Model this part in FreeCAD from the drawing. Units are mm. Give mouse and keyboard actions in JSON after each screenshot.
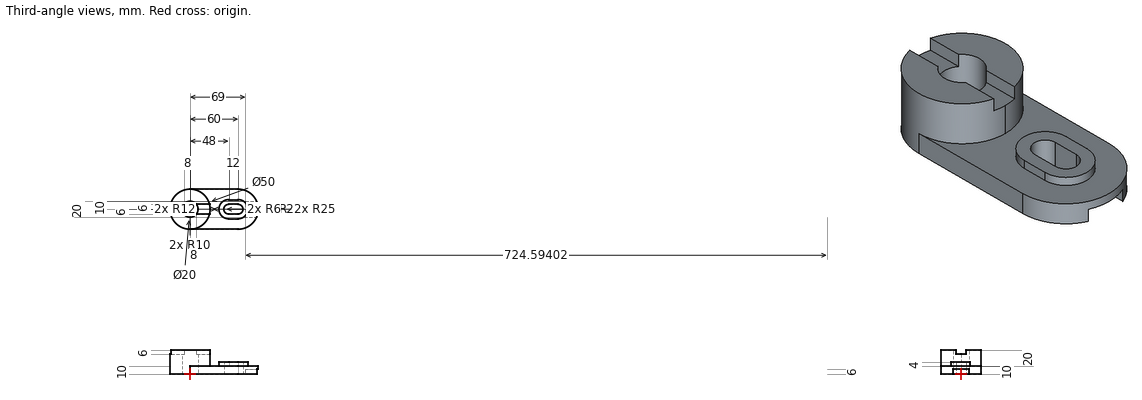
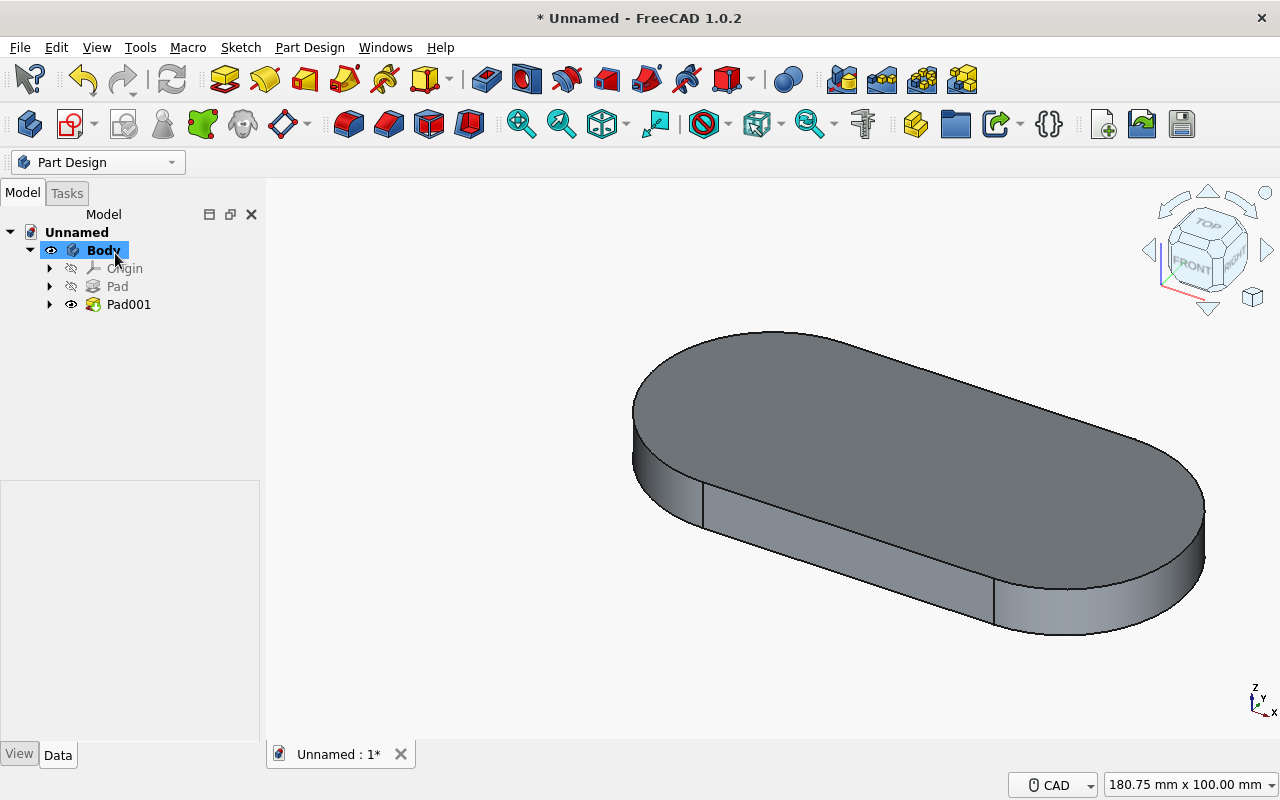
{"action": "left_click", "coordinate": [50, 268]}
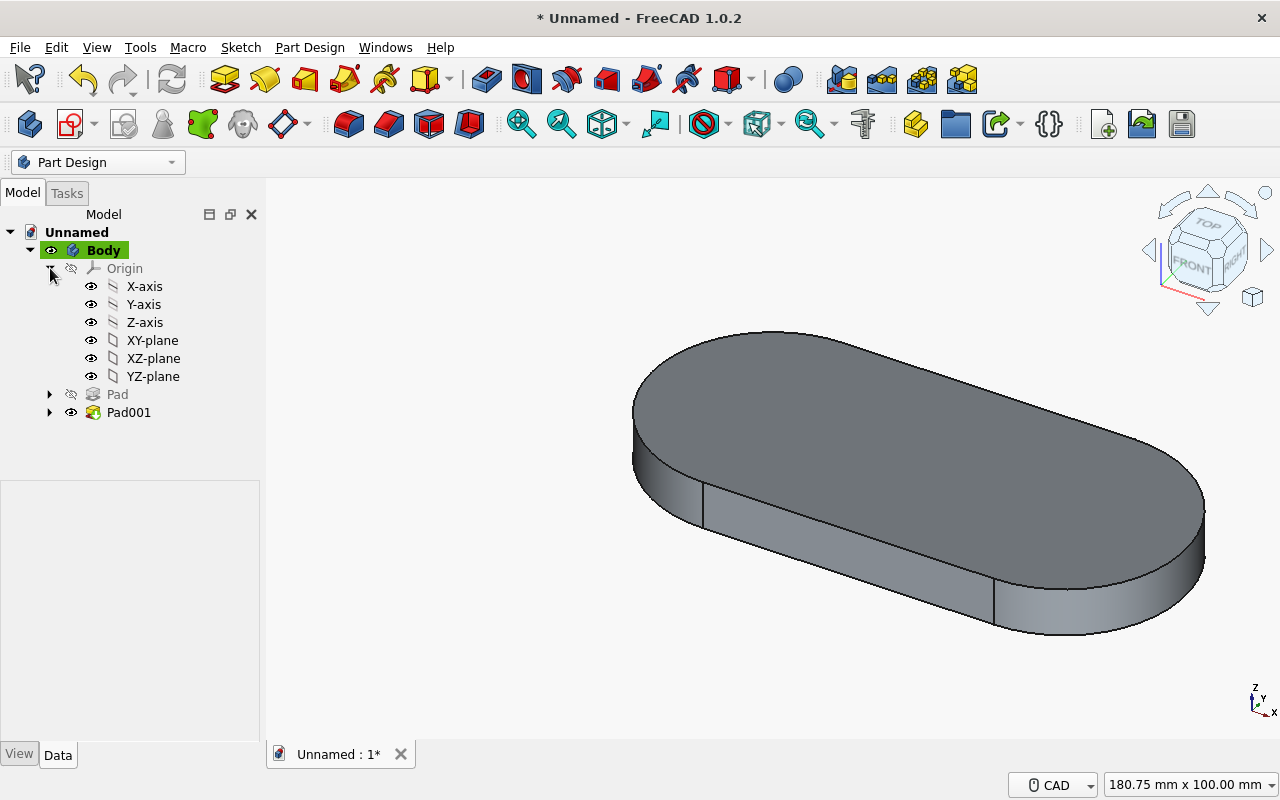
{"action": "left_click", "coordinate": [136, 340]}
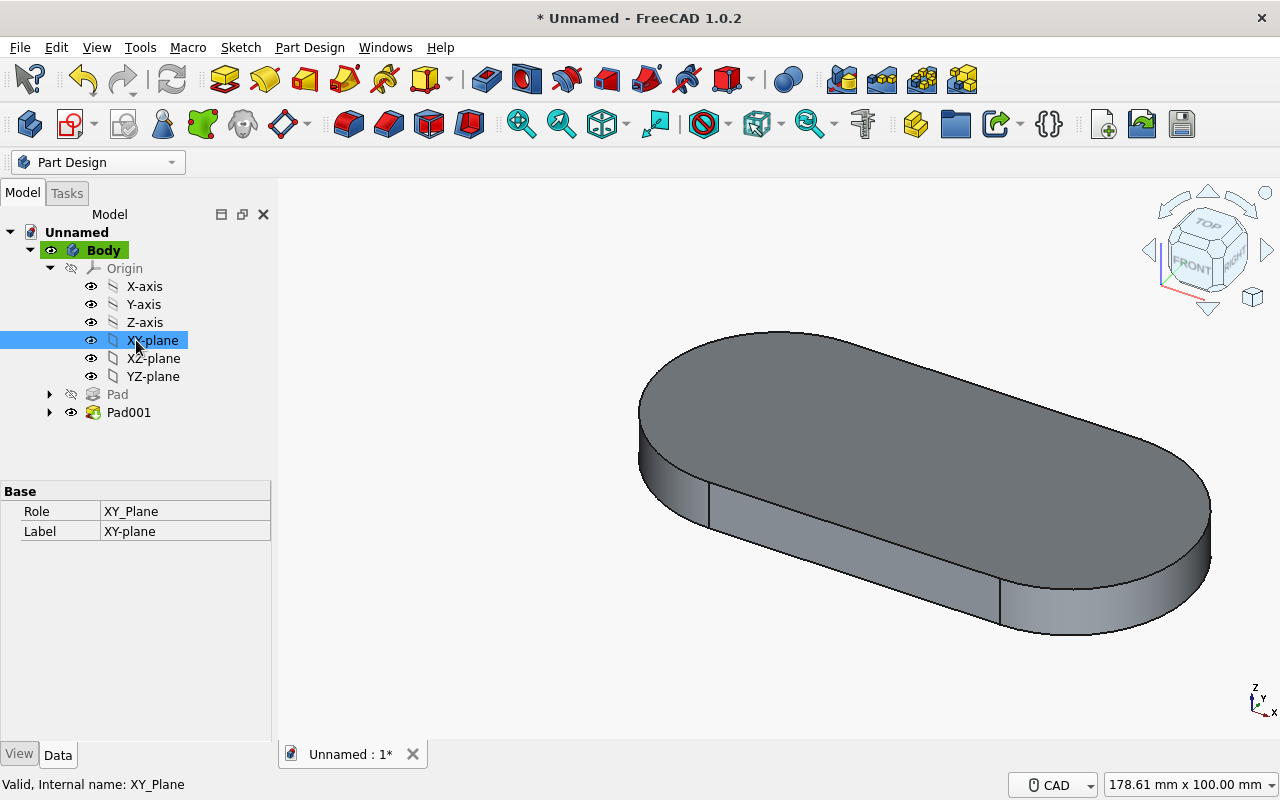
{"action": "left_click", "coordinate": [284, 124]}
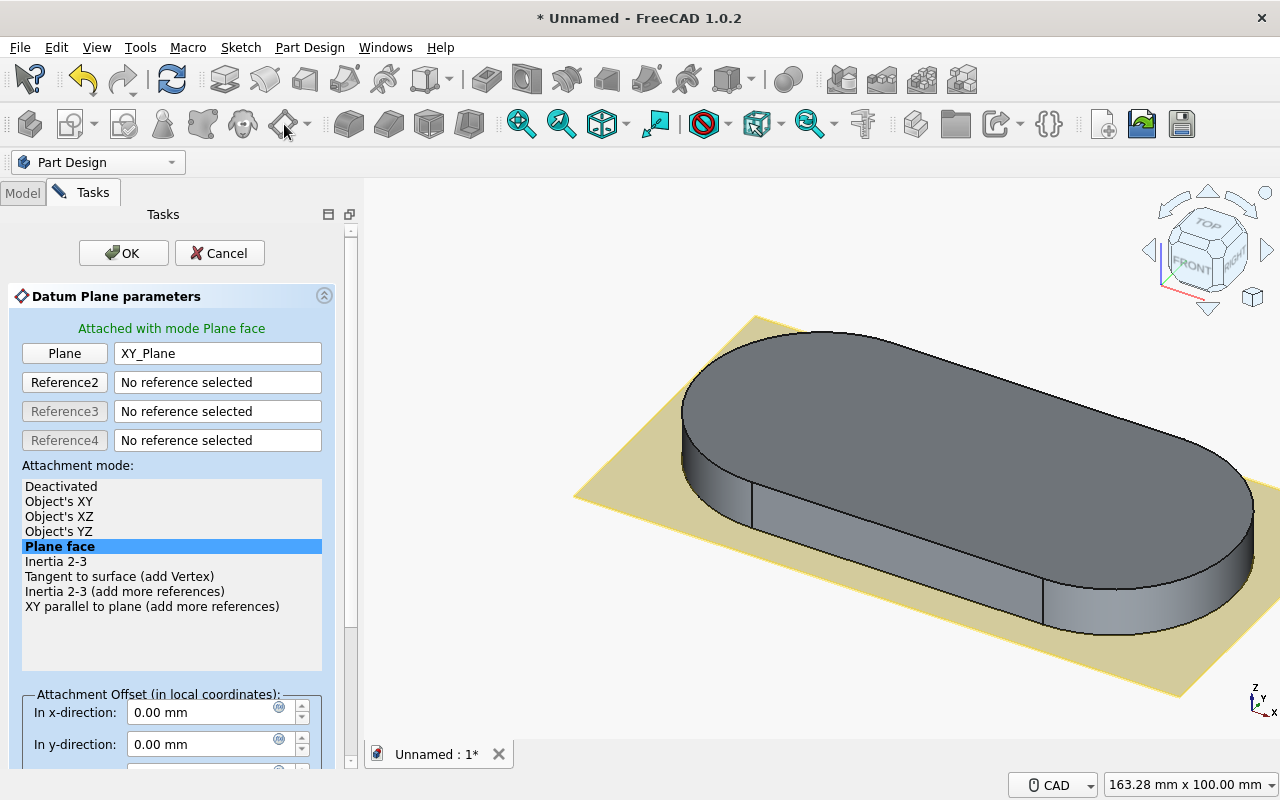
{"action": "scroll", "coordinate": [351, 496], "scroll_direction": "down", "scroll_amount": 2}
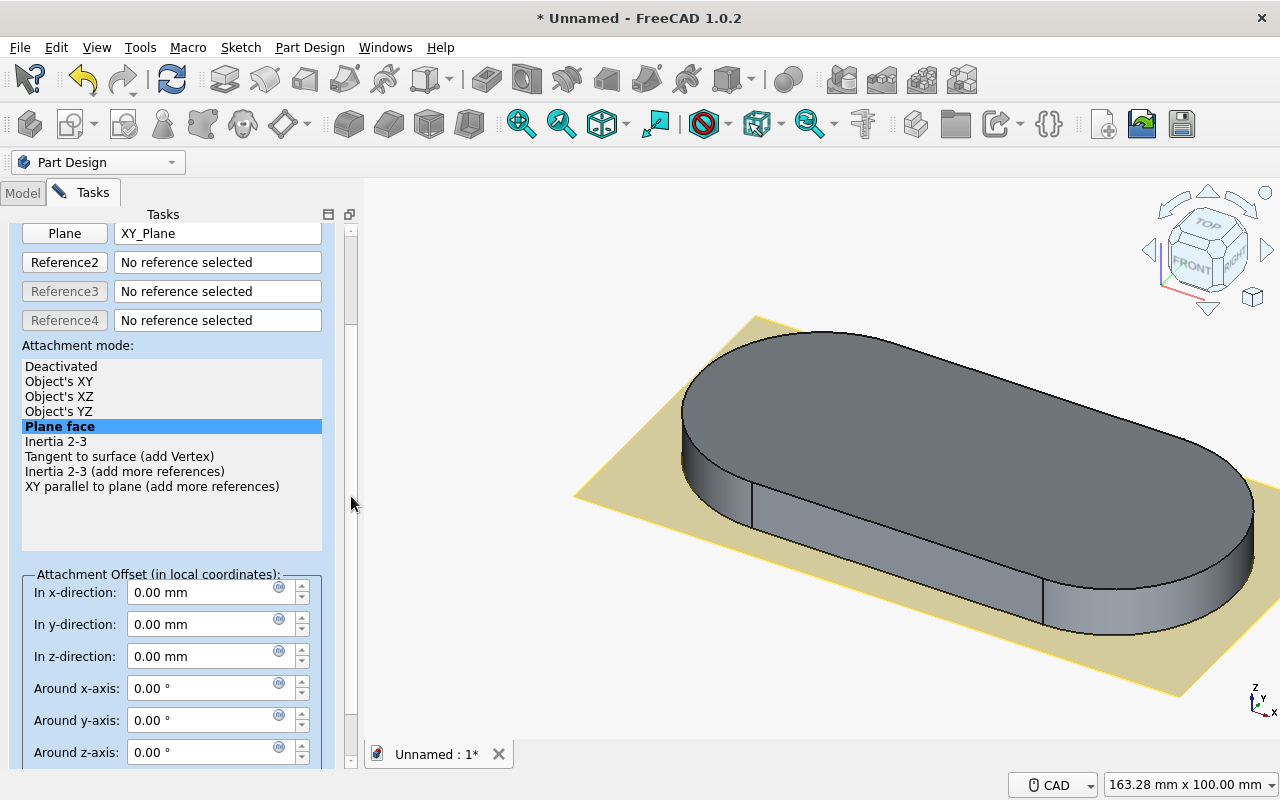
{"action": "triple_click", "coordinate": [210, 656]}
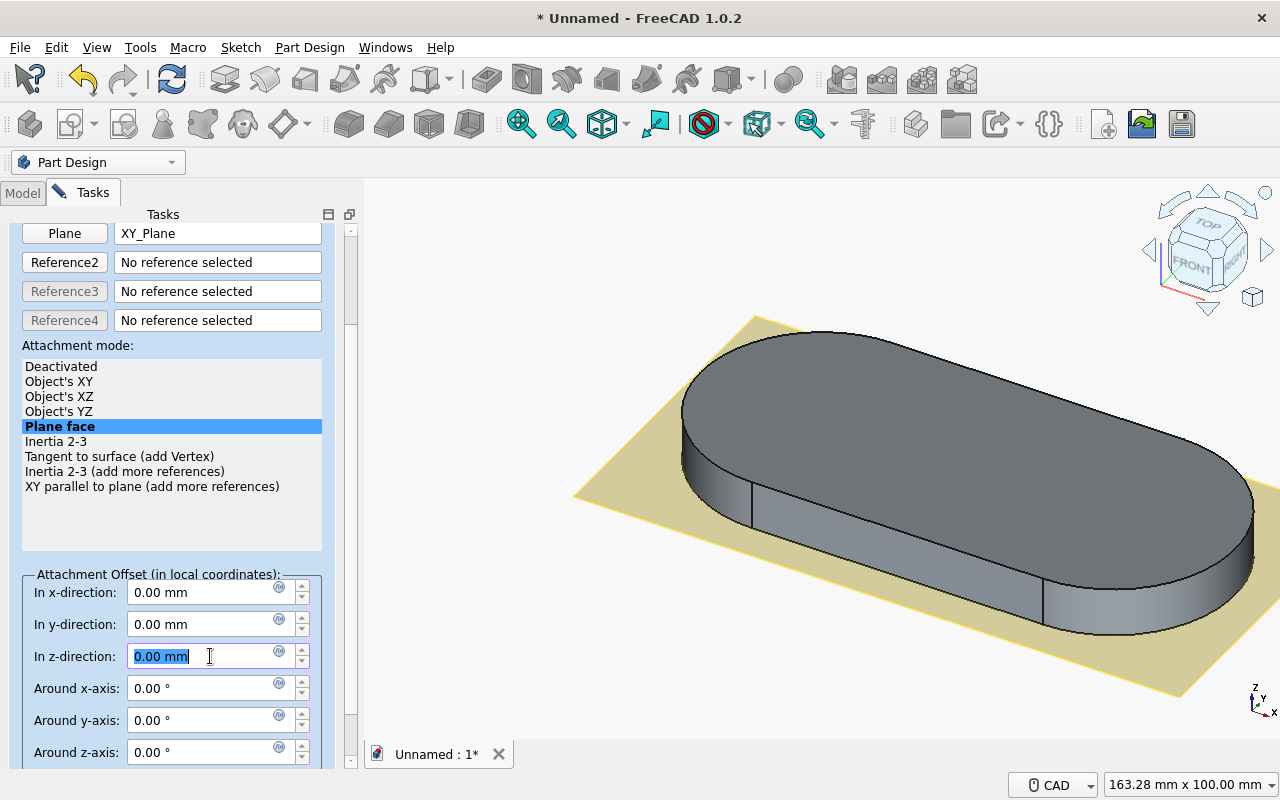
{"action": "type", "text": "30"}
{"action": "key", "text": "Tab"}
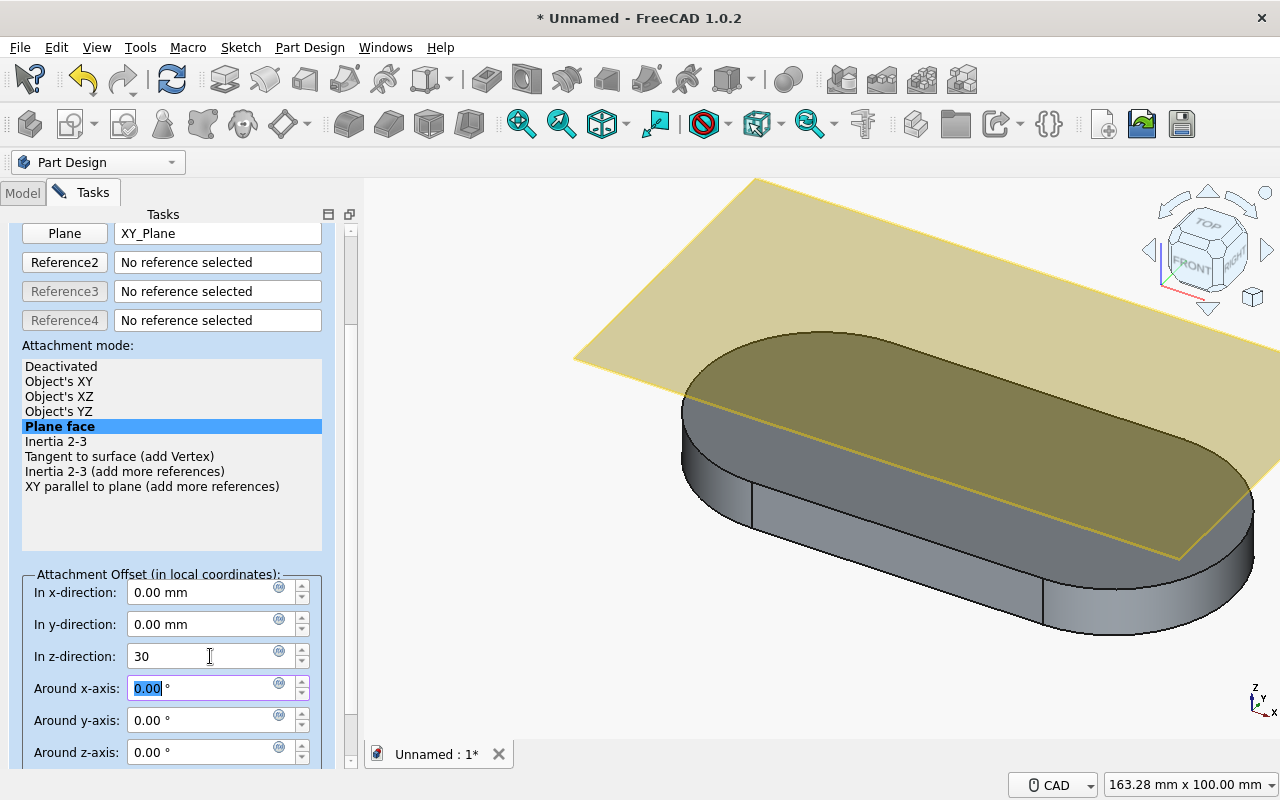
{"action": "scroll", "coordinate": [351, 496], "scroll_direction": "up", "scroll_amount": 3}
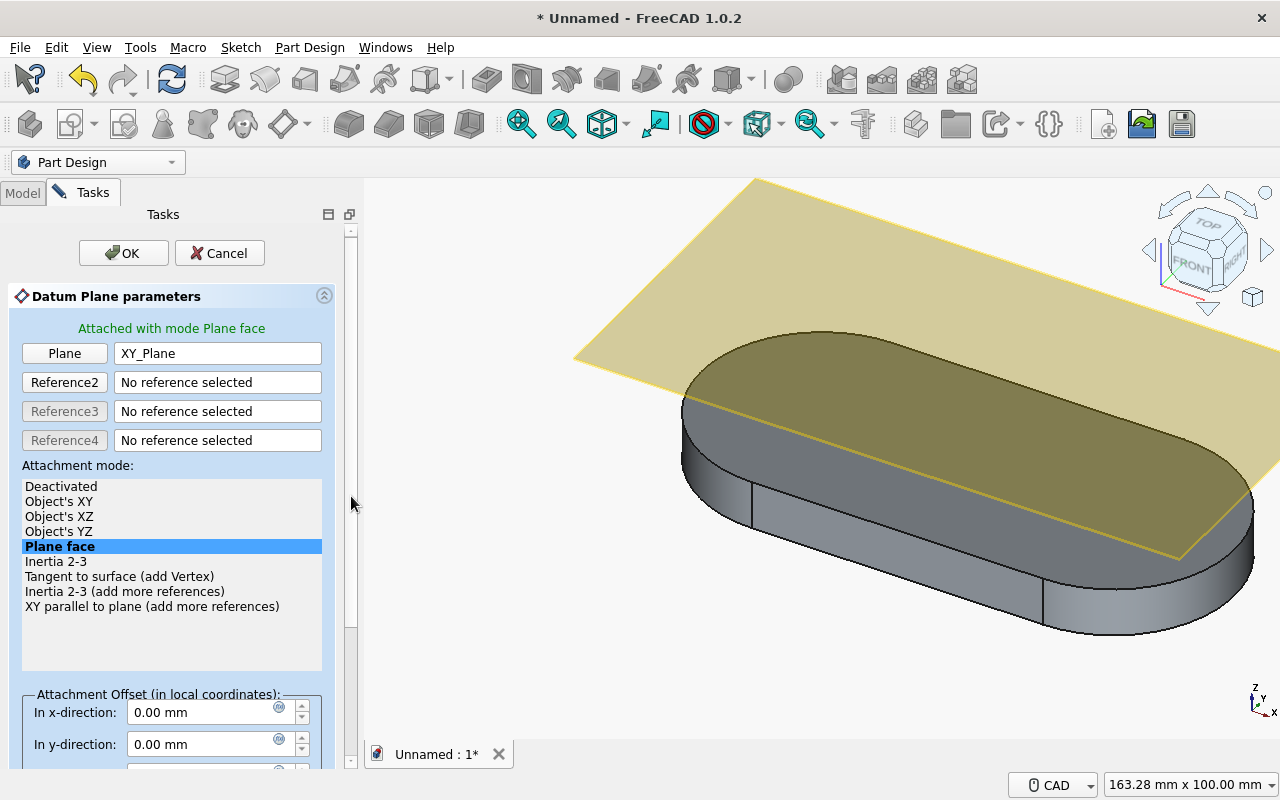
{"action": "left_click", "coordinate": [124, 253]}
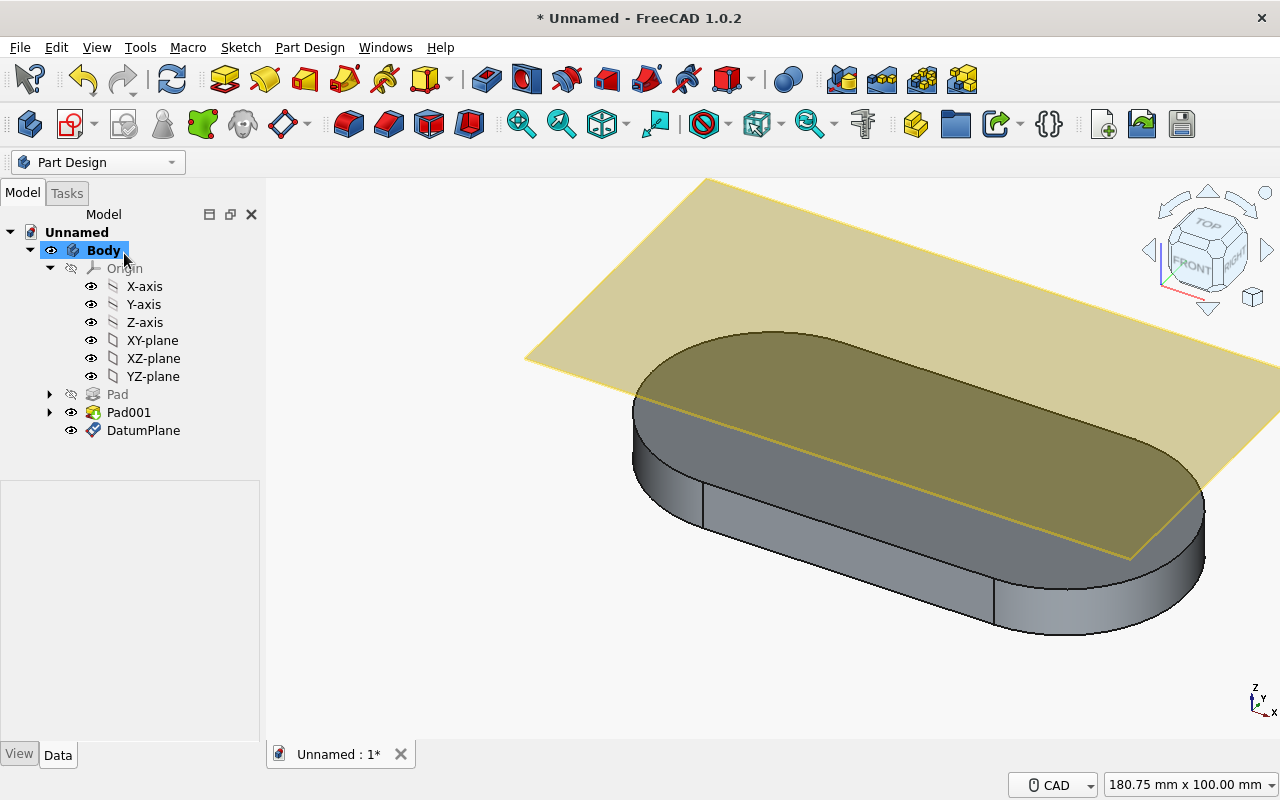
{"action": "left_click", "coordinate": [116, 430]}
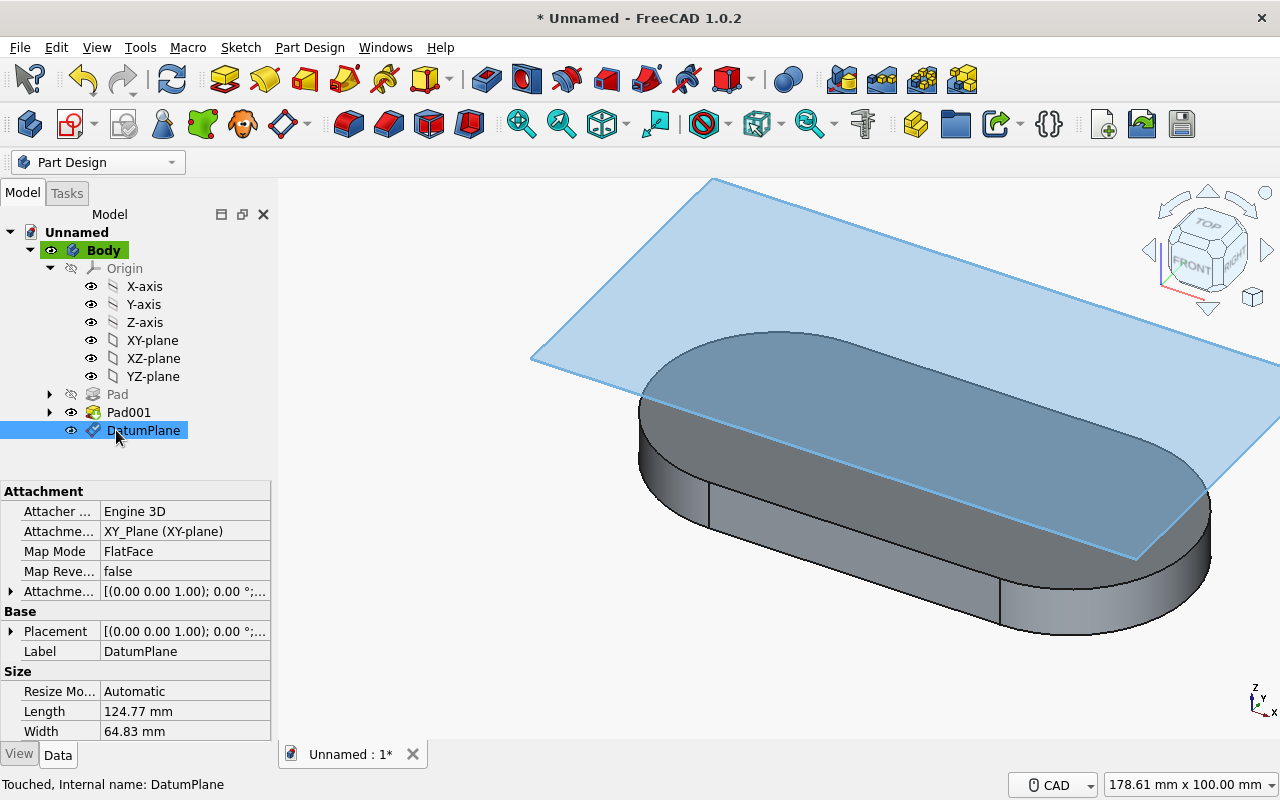
{"action": "left_click", "coordinate": [70, 124]}